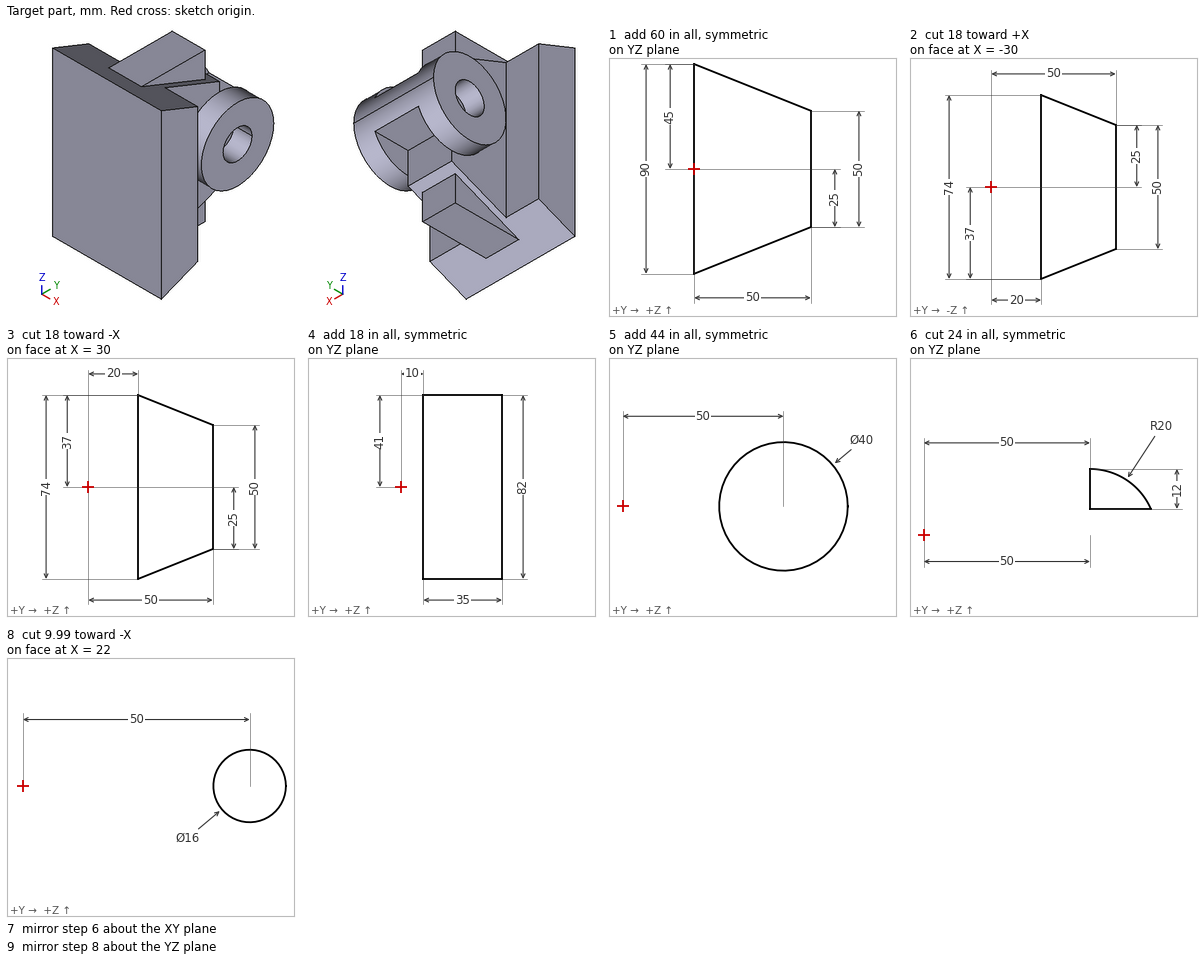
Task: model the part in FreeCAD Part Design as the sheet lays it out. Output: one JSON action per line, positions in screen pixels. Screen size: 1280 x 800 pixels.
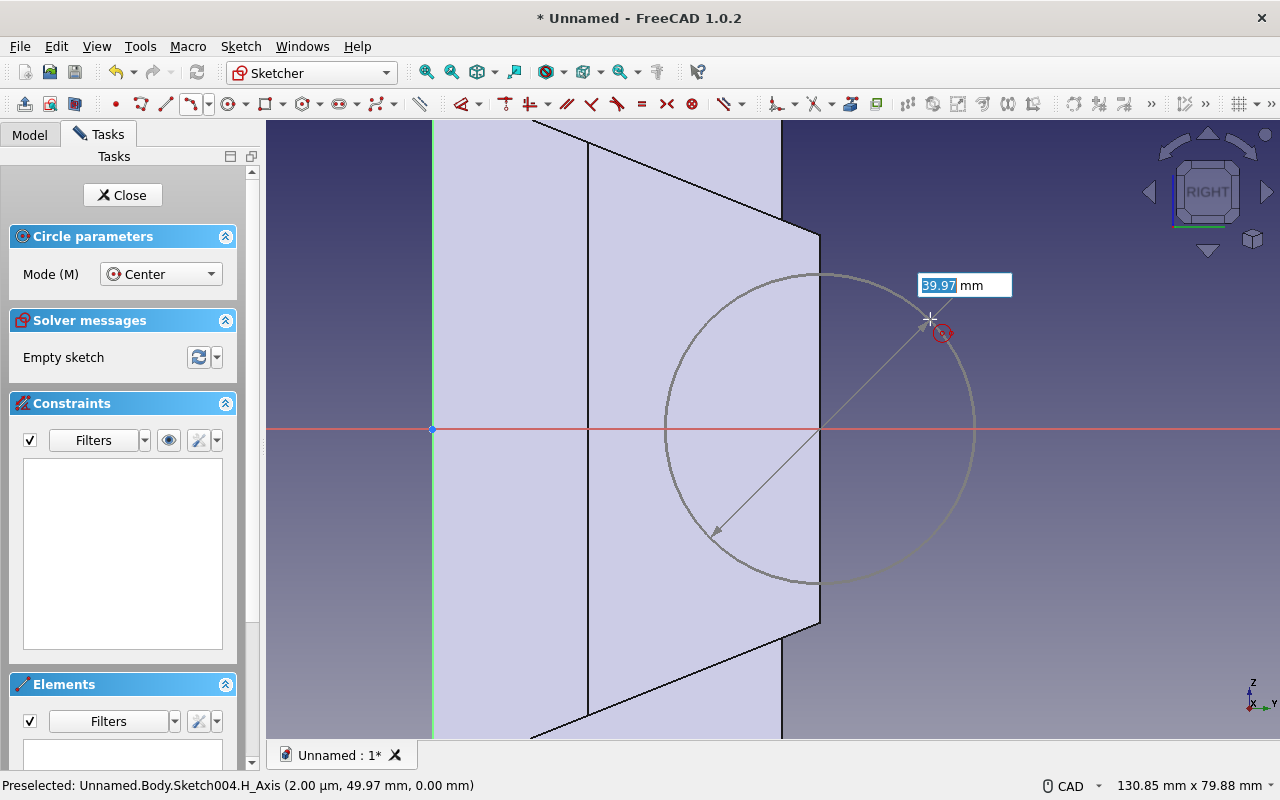
{"action": "type", "text": "40"}
{"action": "key", "text": "Return"}
{"action": "key", "text": "Escape"}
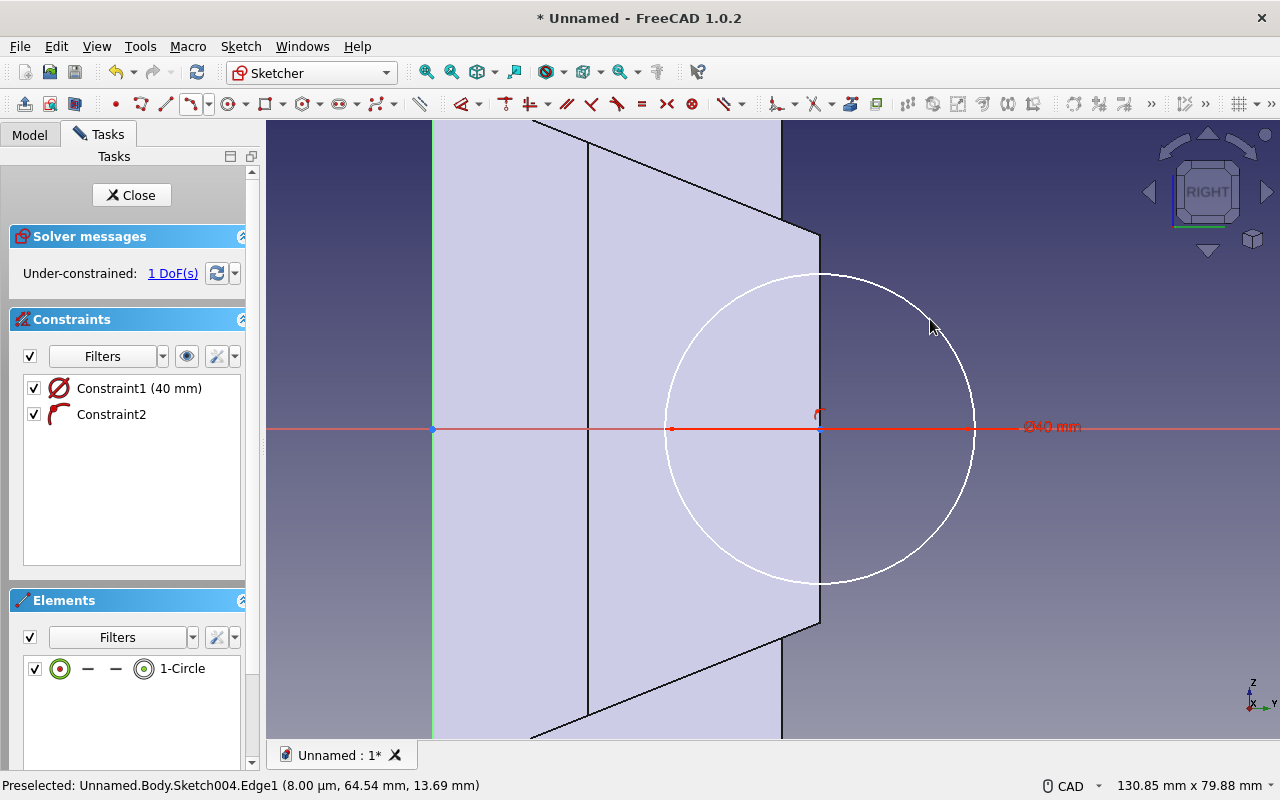
{"action": "left_click", "coordinate": [460, 104]}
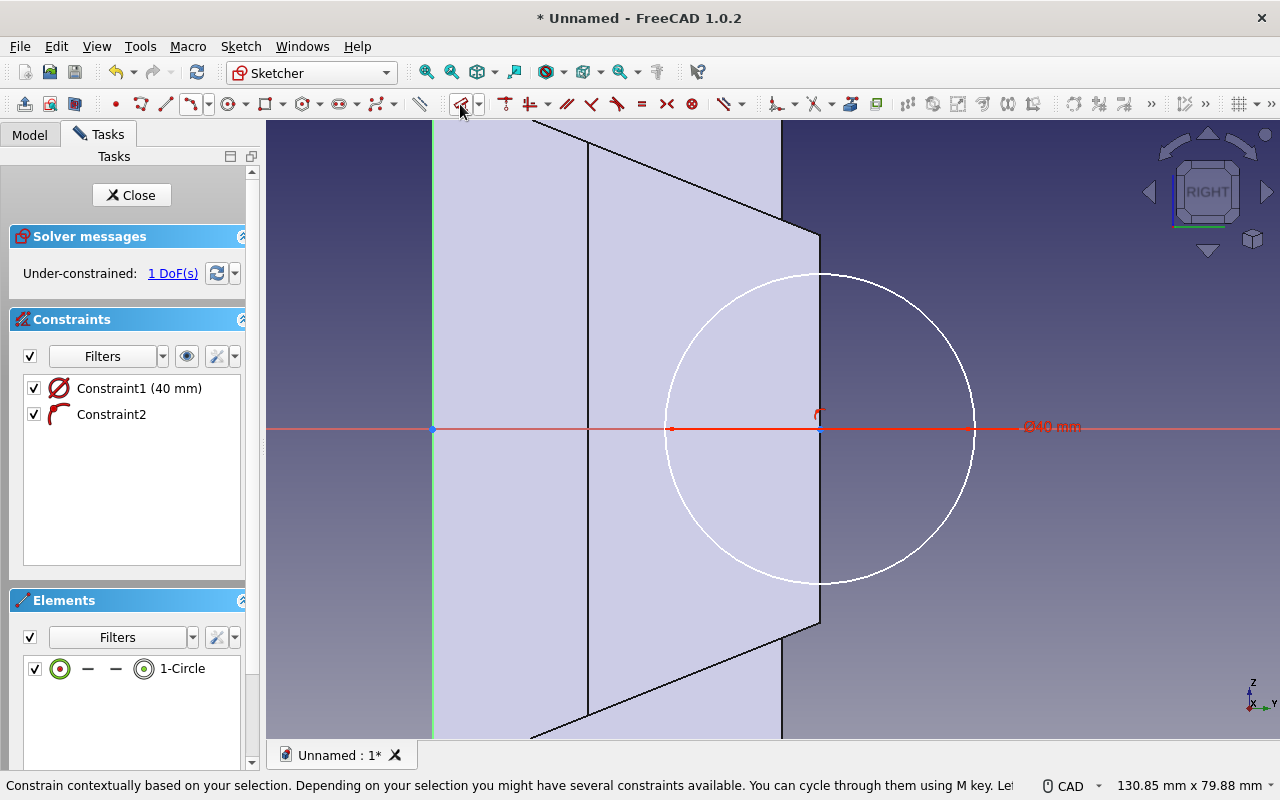
{"action": "left_click", "coordinate": [820, 429]}
{"action": "left_click", "coordinate": [626, 463]}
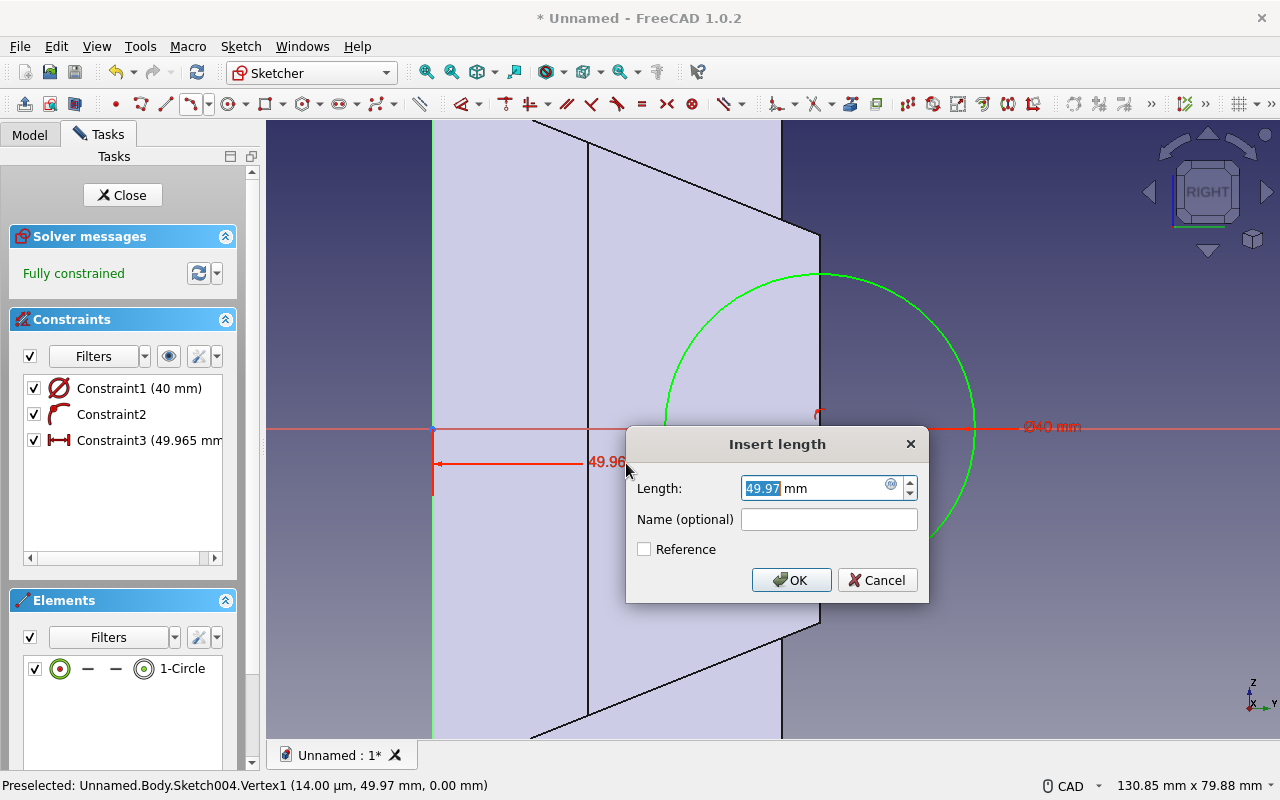
{"action": "type", "text": "50"}
{"action": "key", "text": "Return"}
{"action": "key", "text": "Escape"}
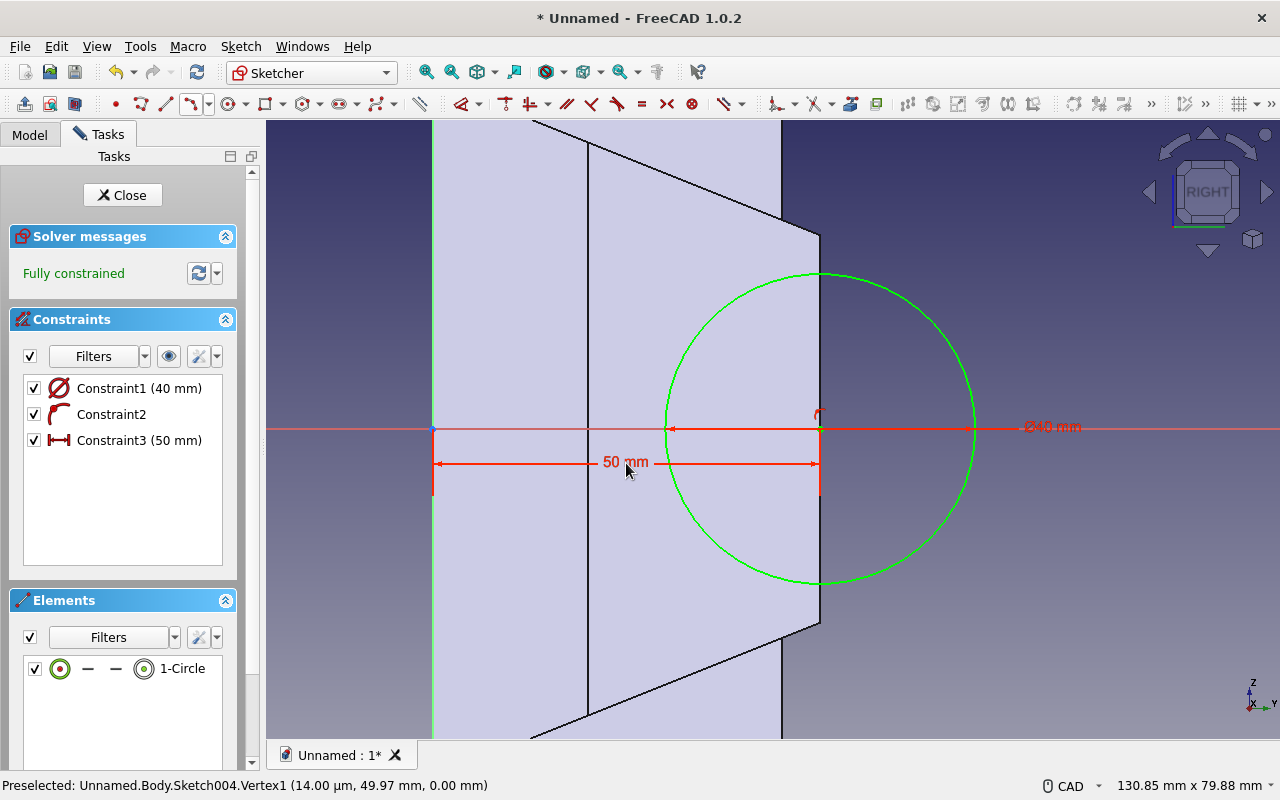
{"action": "left_click", "coordinate": [123, 195]}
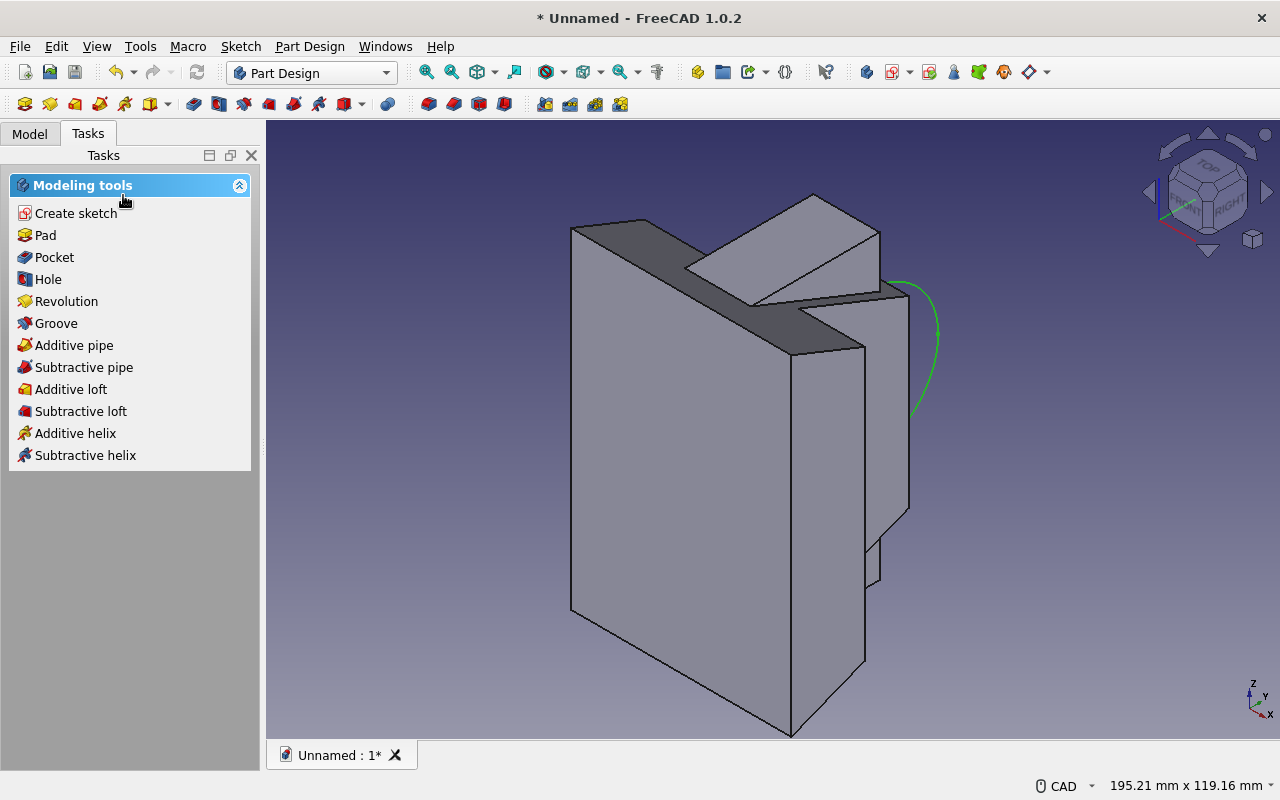
{"action": "left_click", "coordinate": [25, 104]}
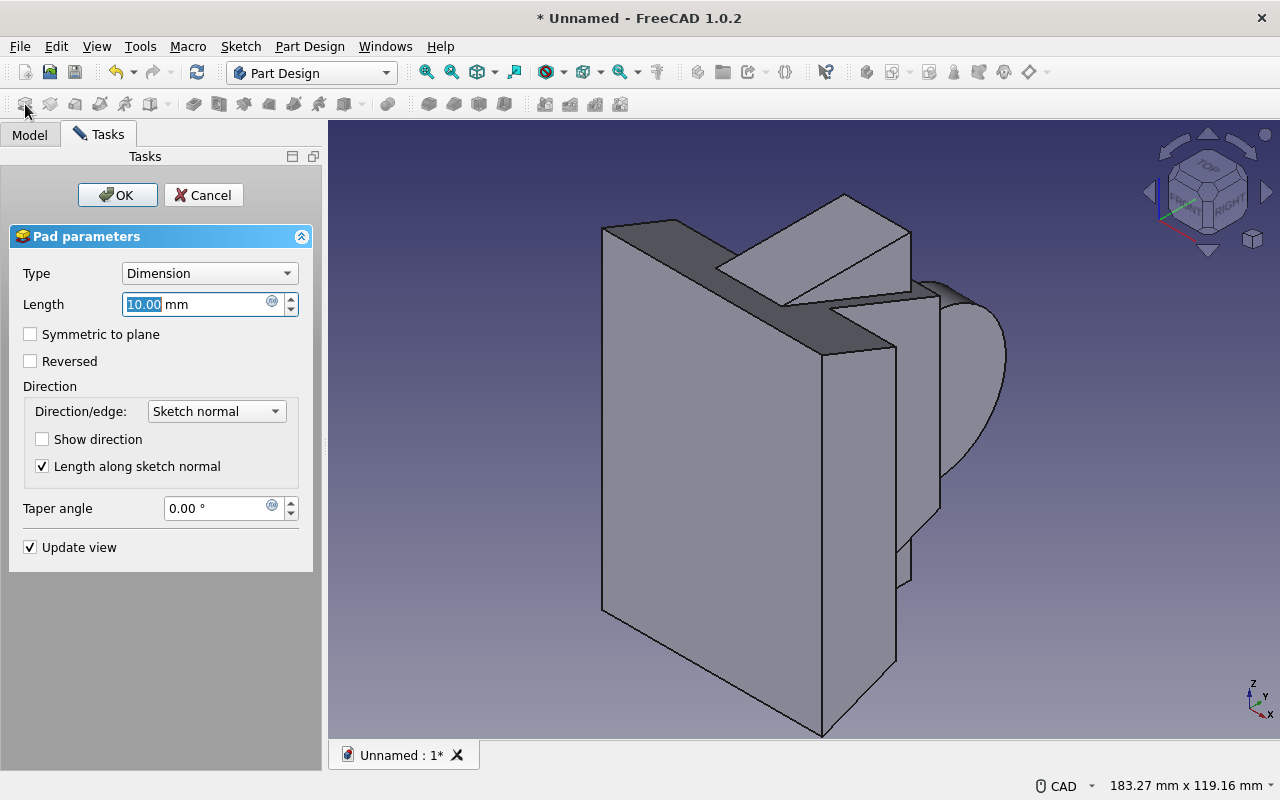
{"action": "type", "text": "44"}
{"action": "key", "text": "Tab"}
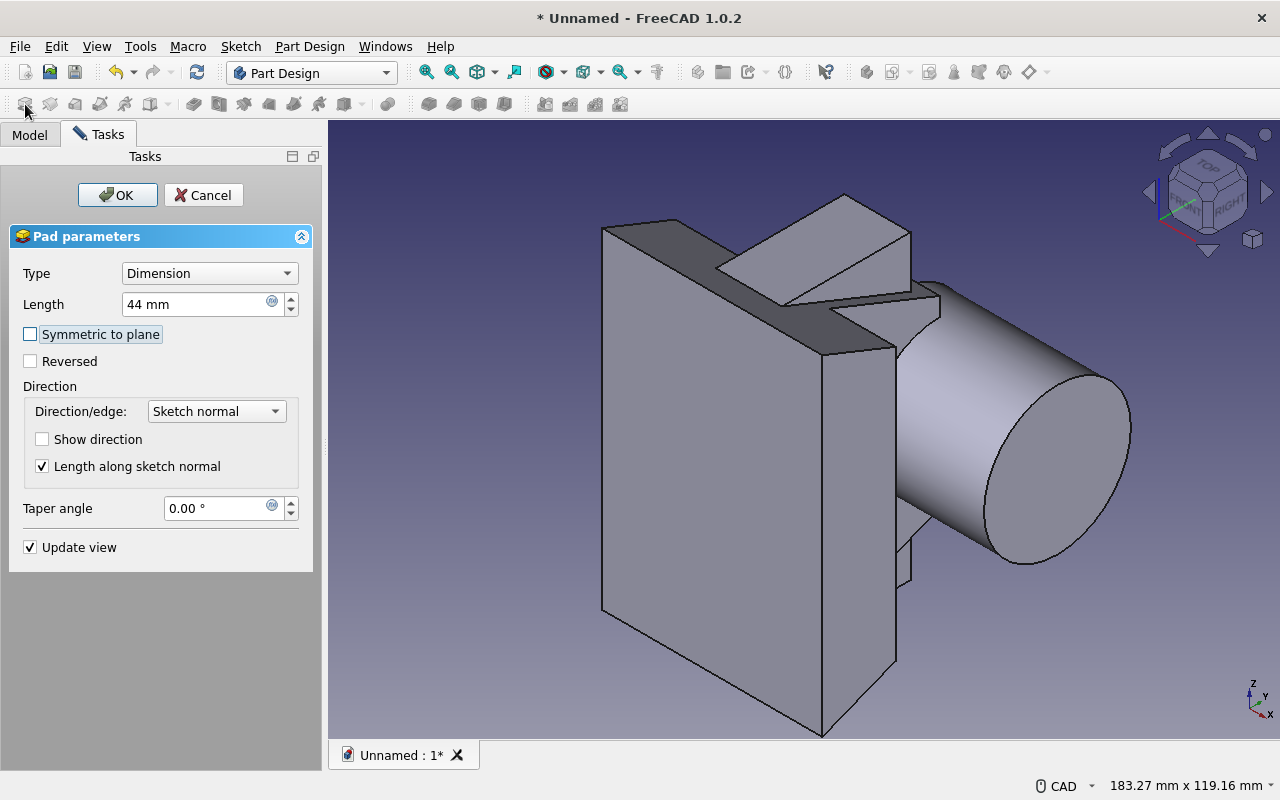
{"action": "left_click", "coordinate": [31, 334]}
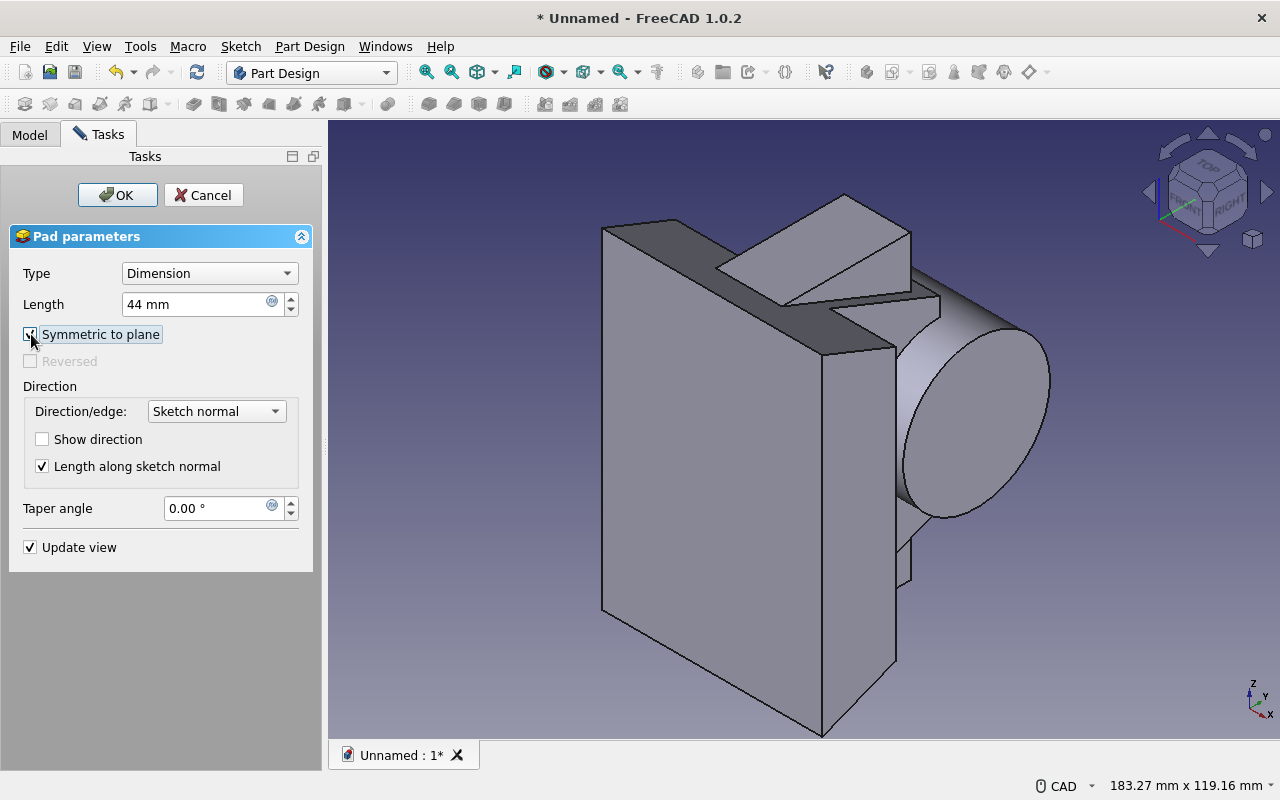
{"action": "left_click", "coordinate": [118, 195]}